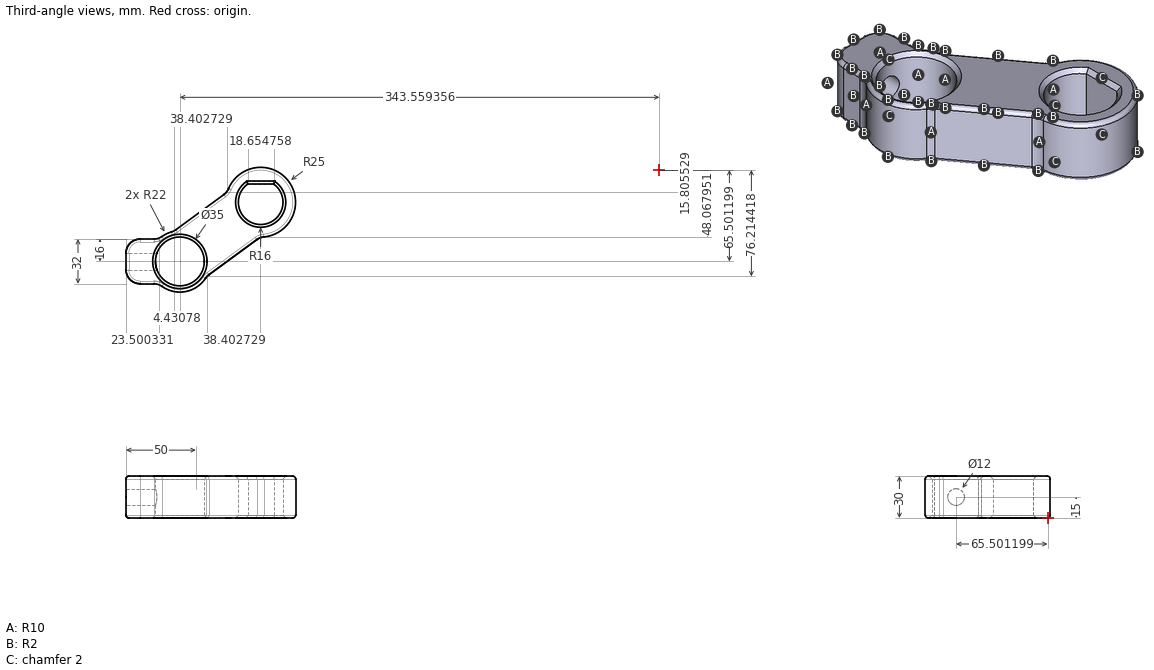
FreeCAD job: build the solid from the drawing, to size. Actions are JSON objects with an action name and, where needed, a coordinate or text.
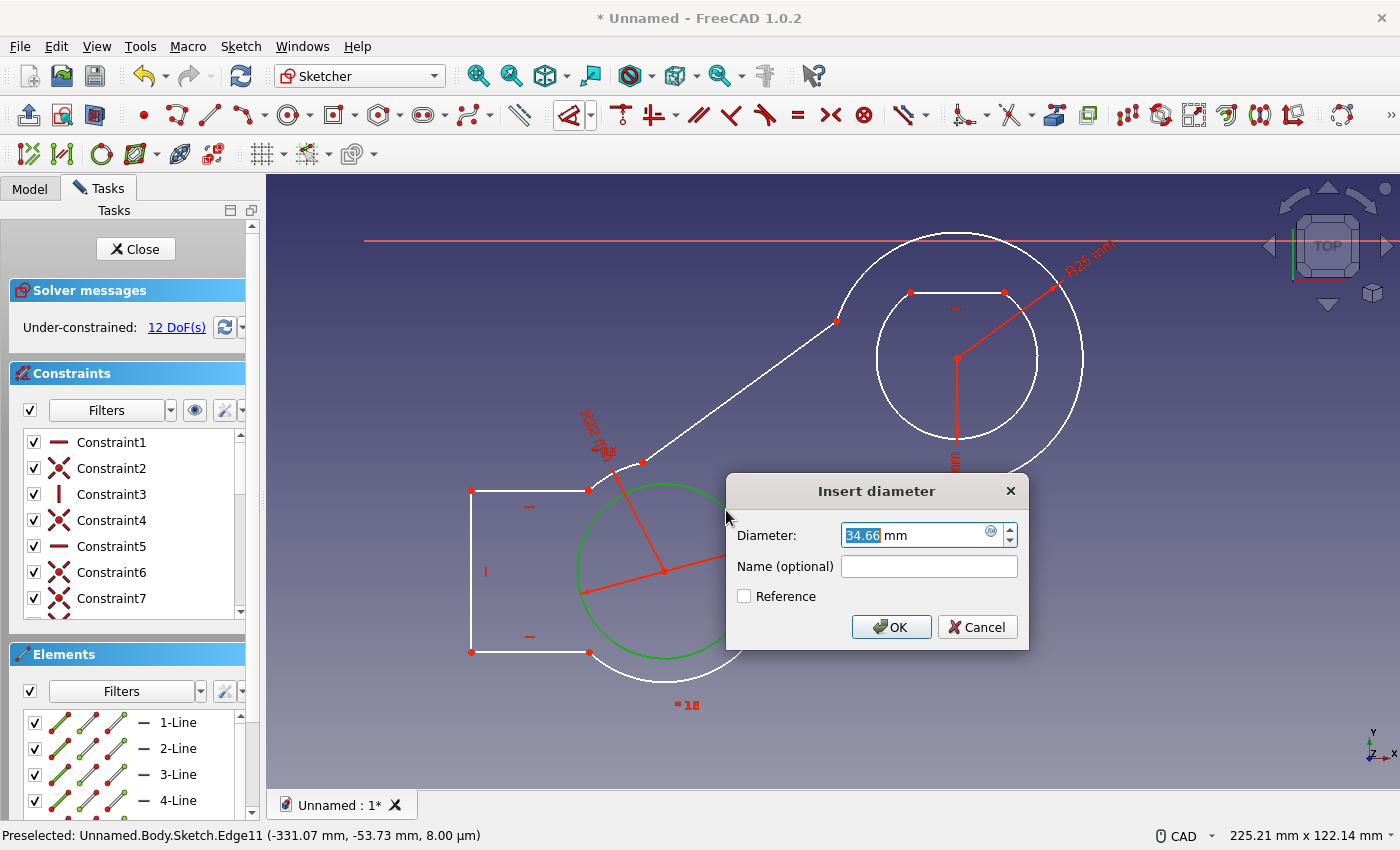
{"action": "type", "text": "35"}
{"action": "key", "text": "Return"}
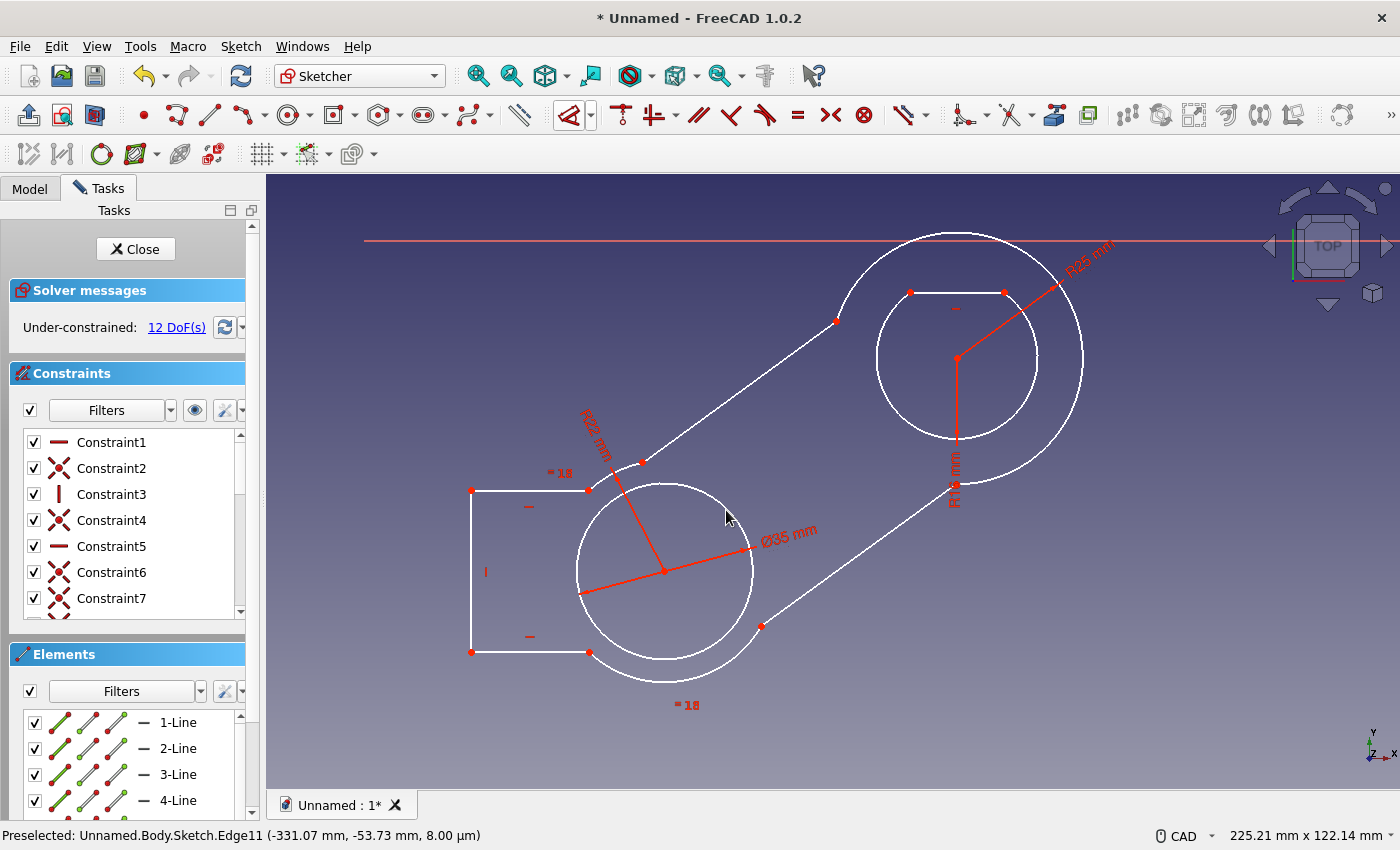
{"action": "left_click", "coordinate": [471, 539]}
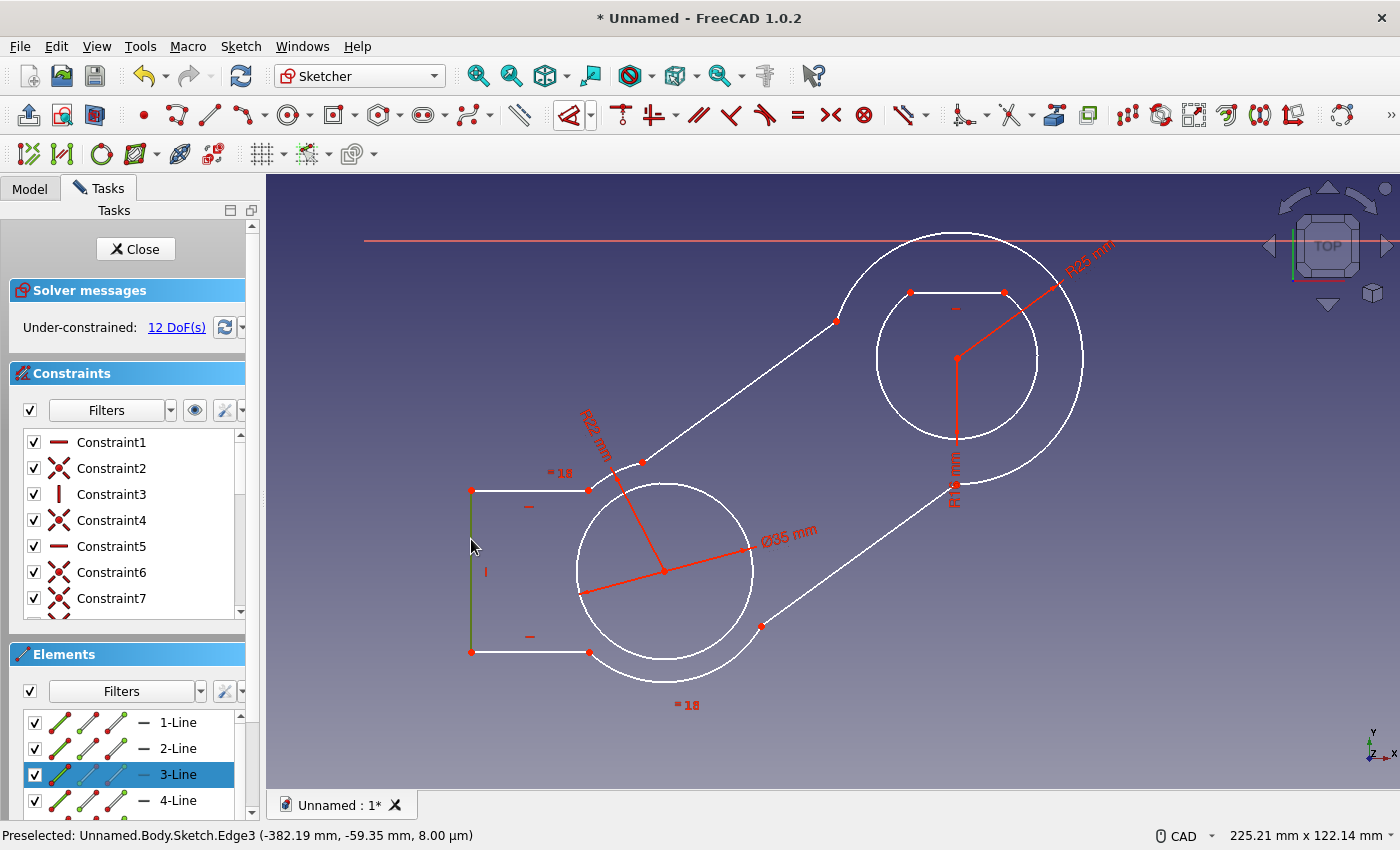
{"action": "left_click", "coordinate": [590, 116]}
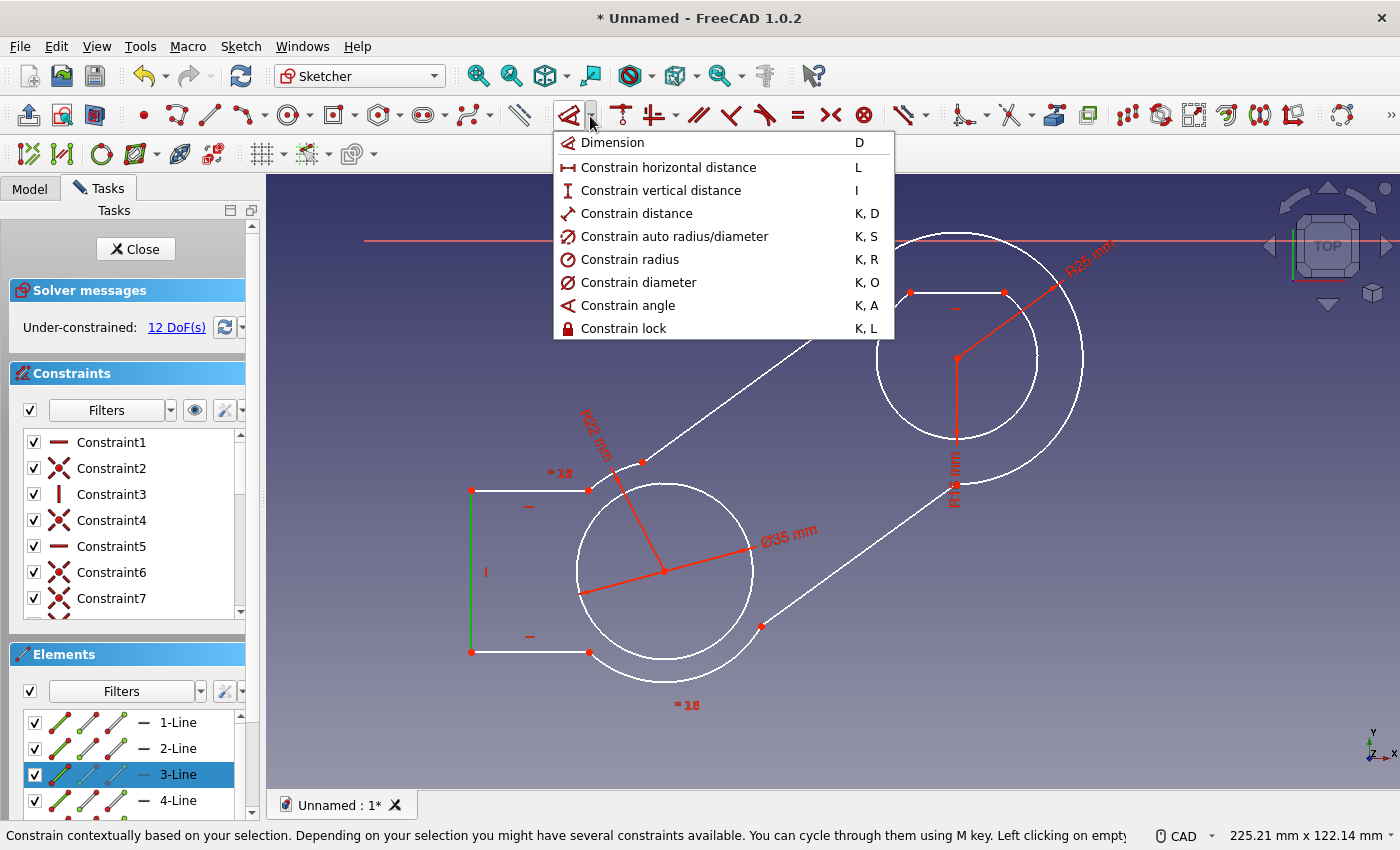
{"action": "left_click", "coordinate": [724, 190]}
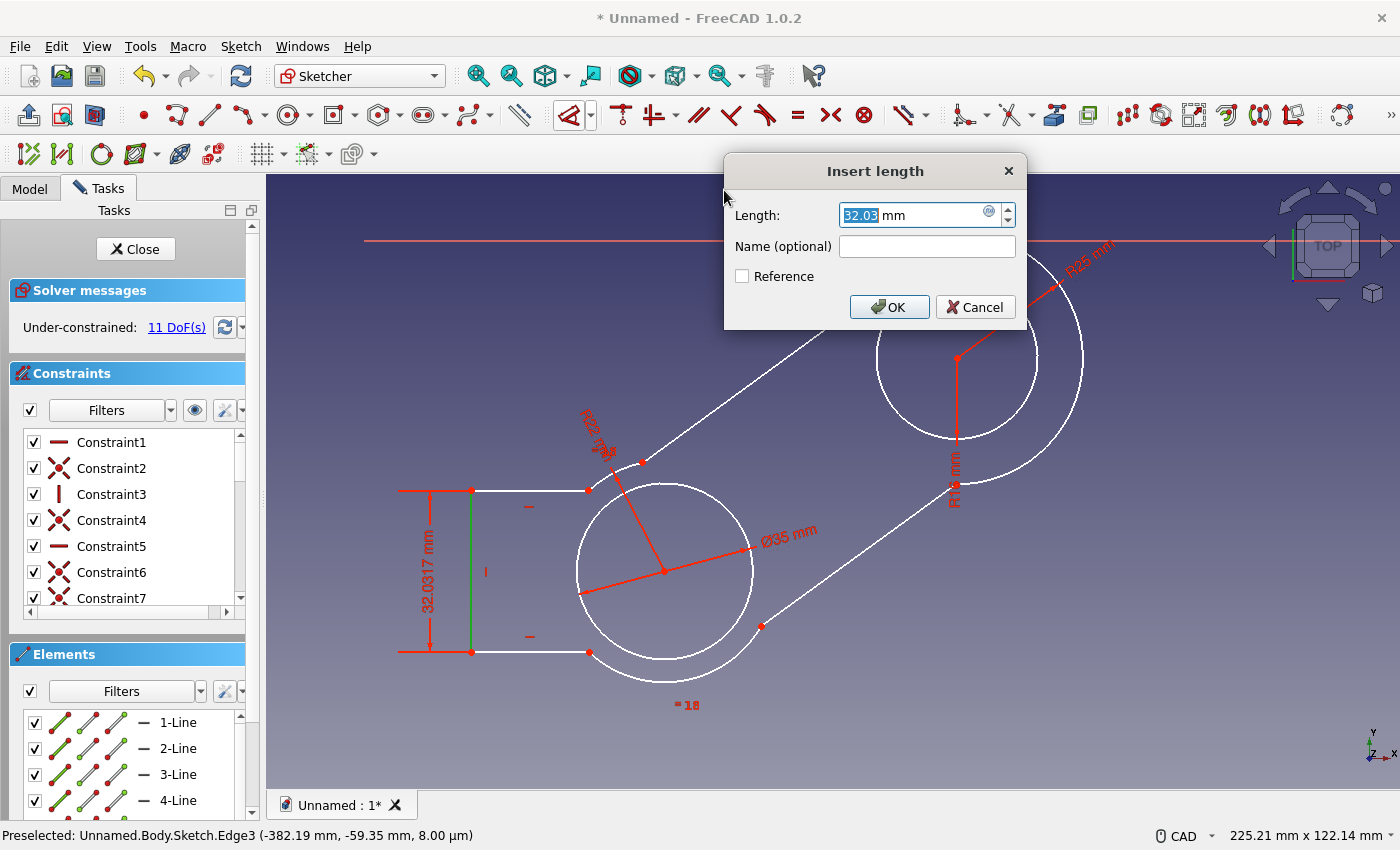
{"action": "type", "text": "32"}
{"action": "key", "text": "Return"}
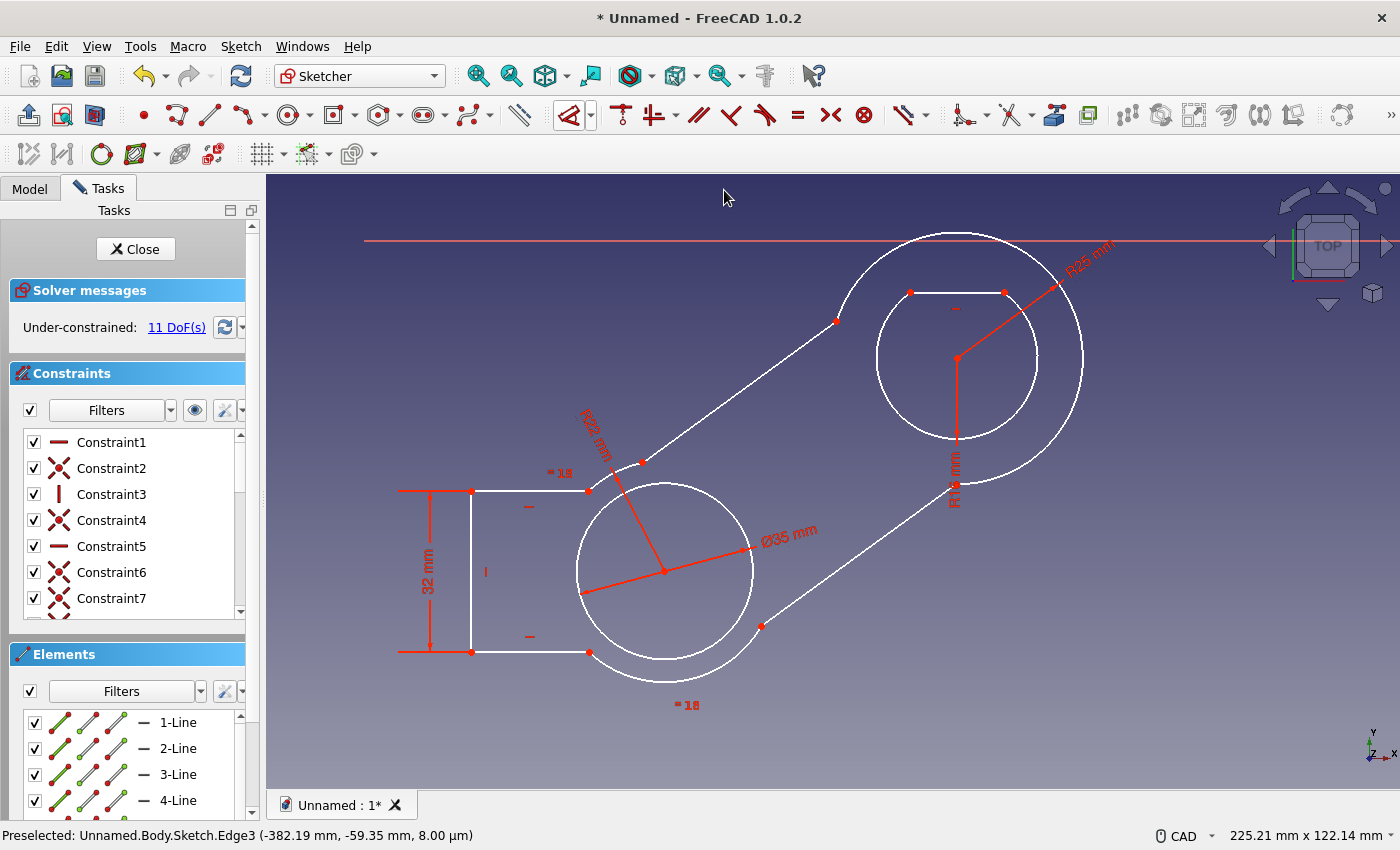
{"action": "left_click", "coordinate": [589, 491]}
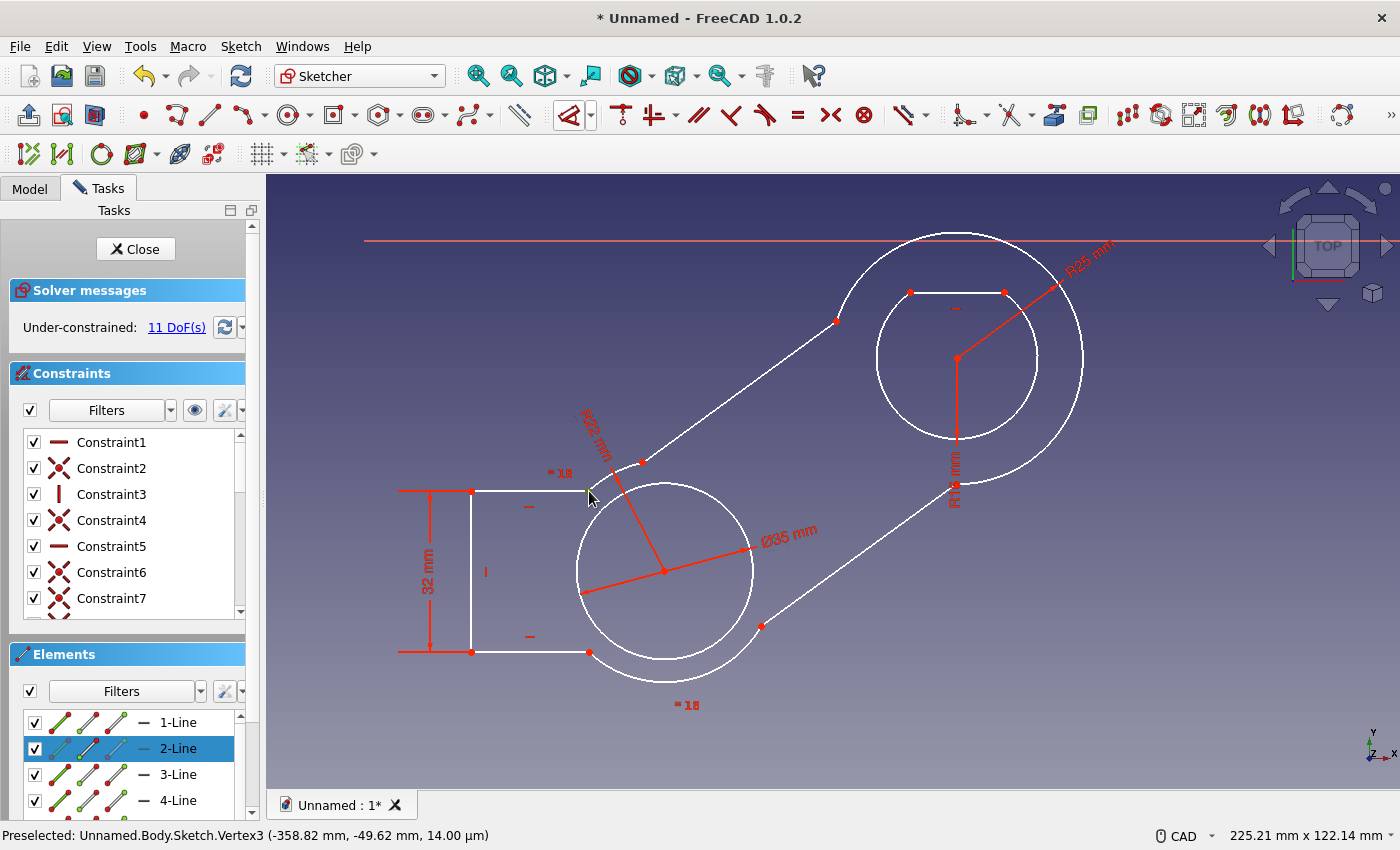
{"action": "left_click", "coordinate": [665, 571]}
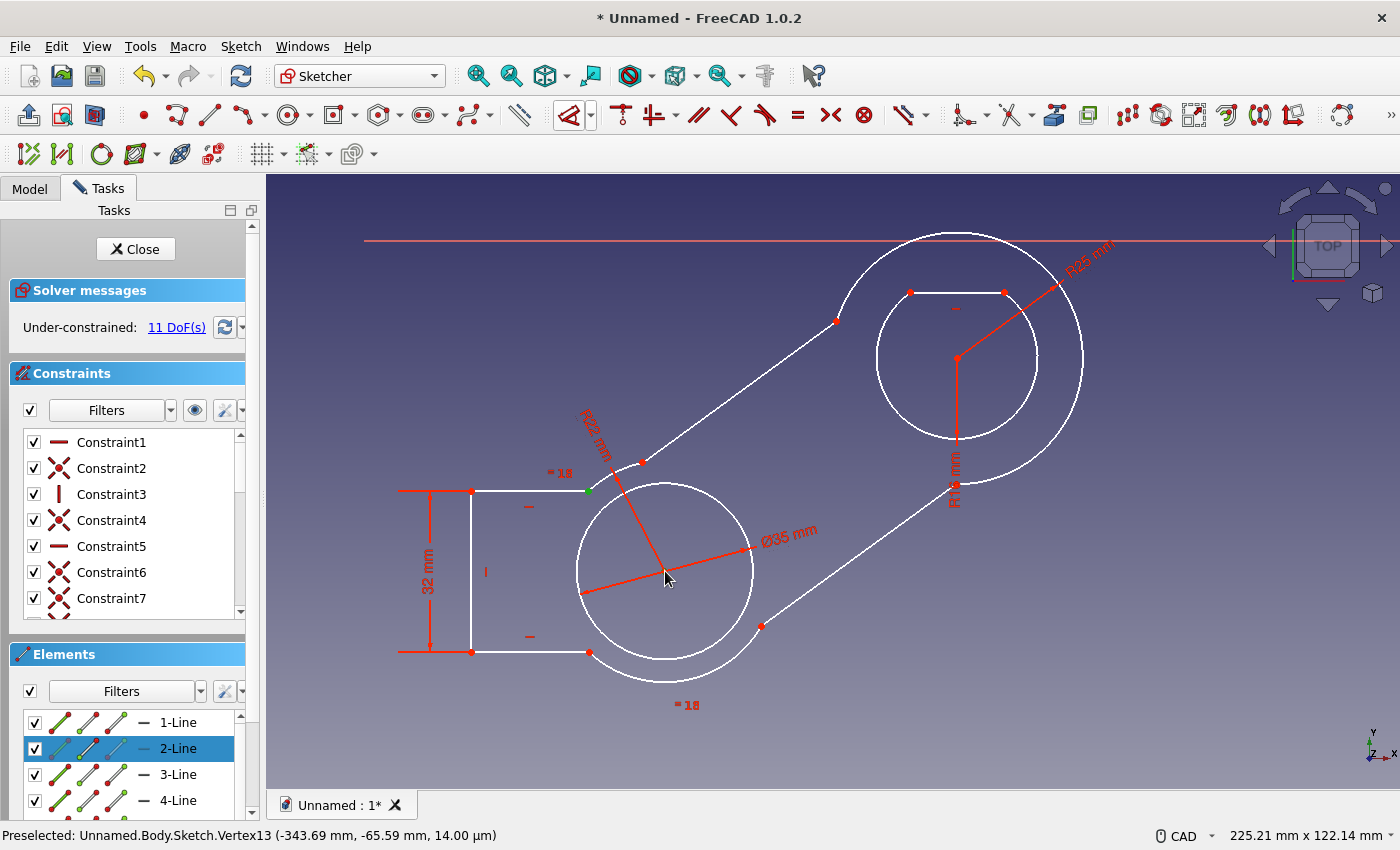
{"action": "key", "text": "i"}